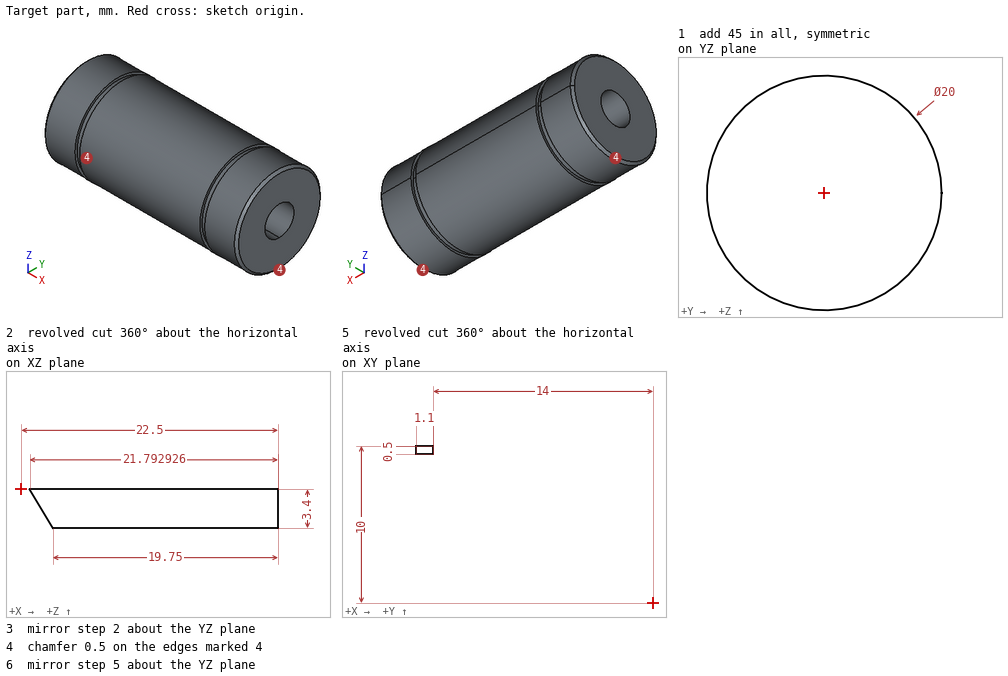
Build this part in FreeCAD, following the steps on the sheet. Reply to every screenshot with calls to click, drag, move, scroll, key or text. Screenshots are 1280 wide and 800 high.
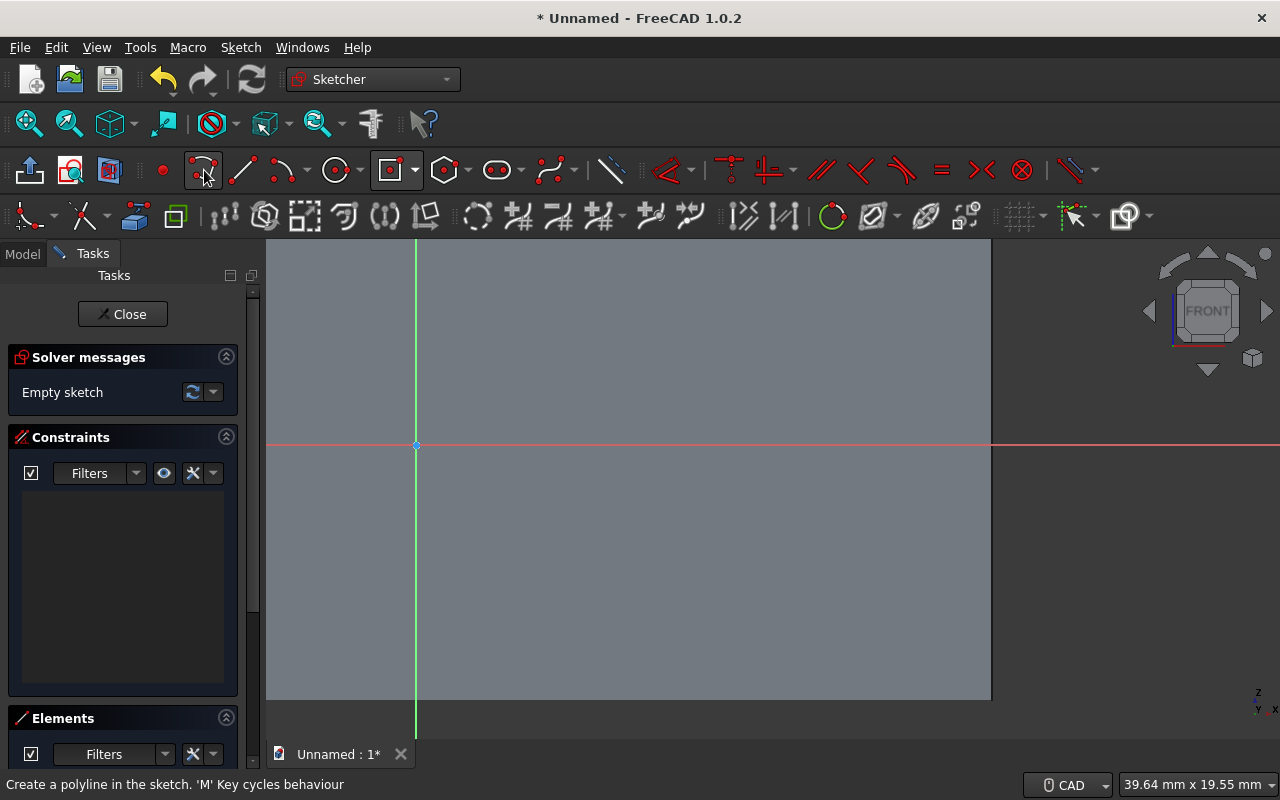
click(434, 445)
click(992, 454)
click(992, 532)
click(486, 532)
click(434, 445)
key(Escape)
key(Escape)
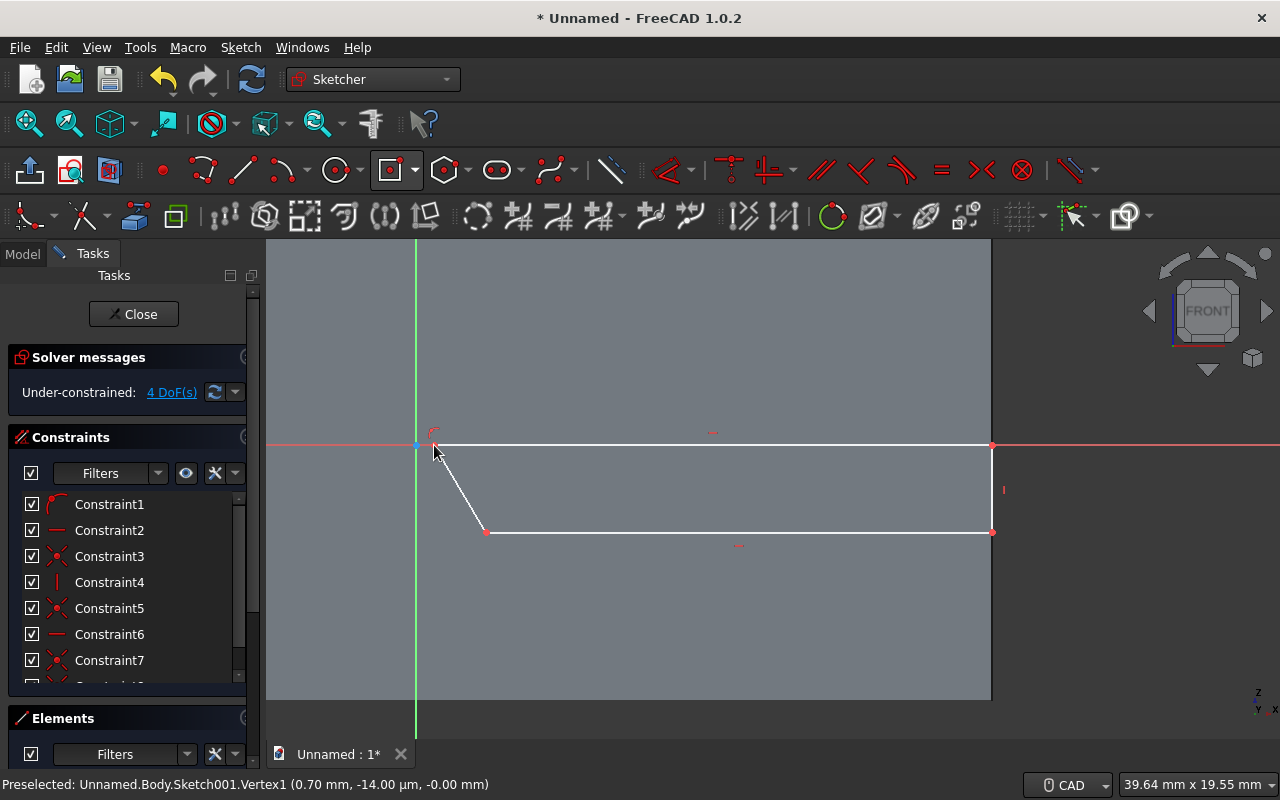
click(992, 471)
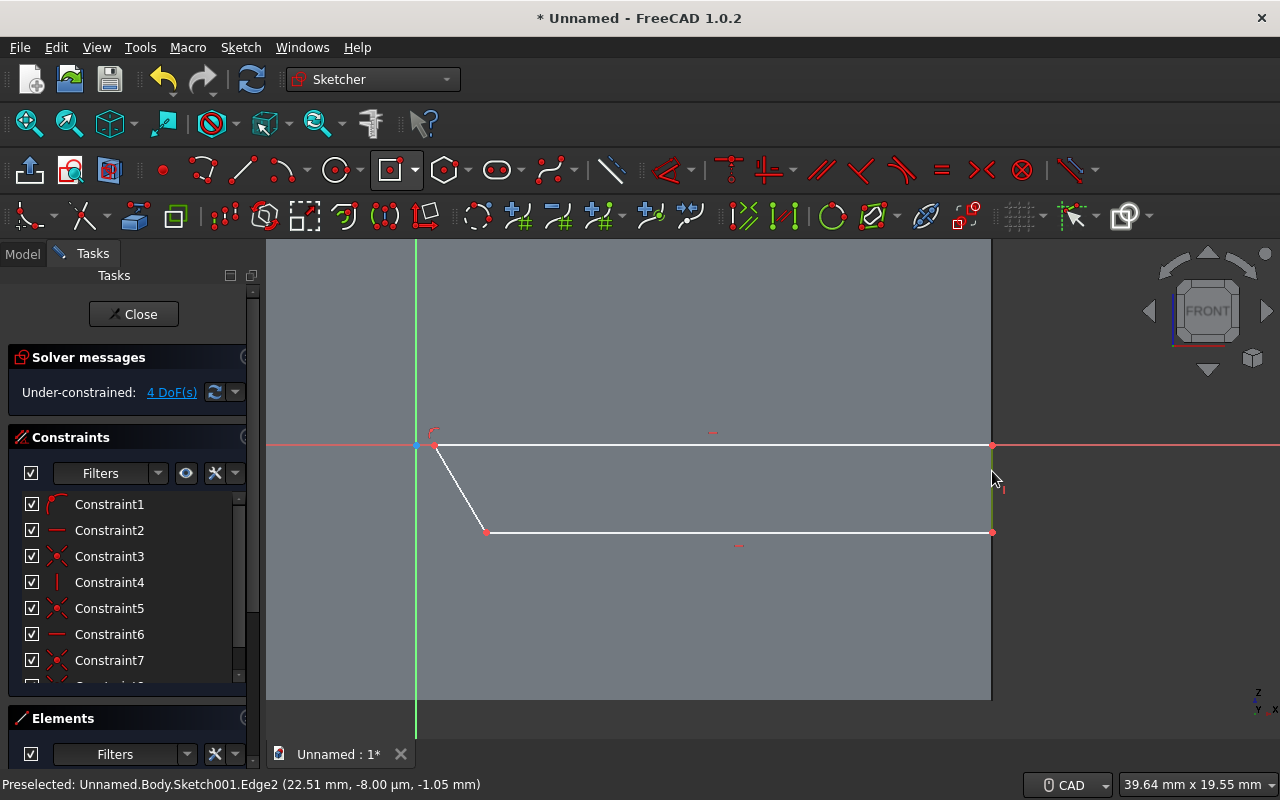
click(694, 170)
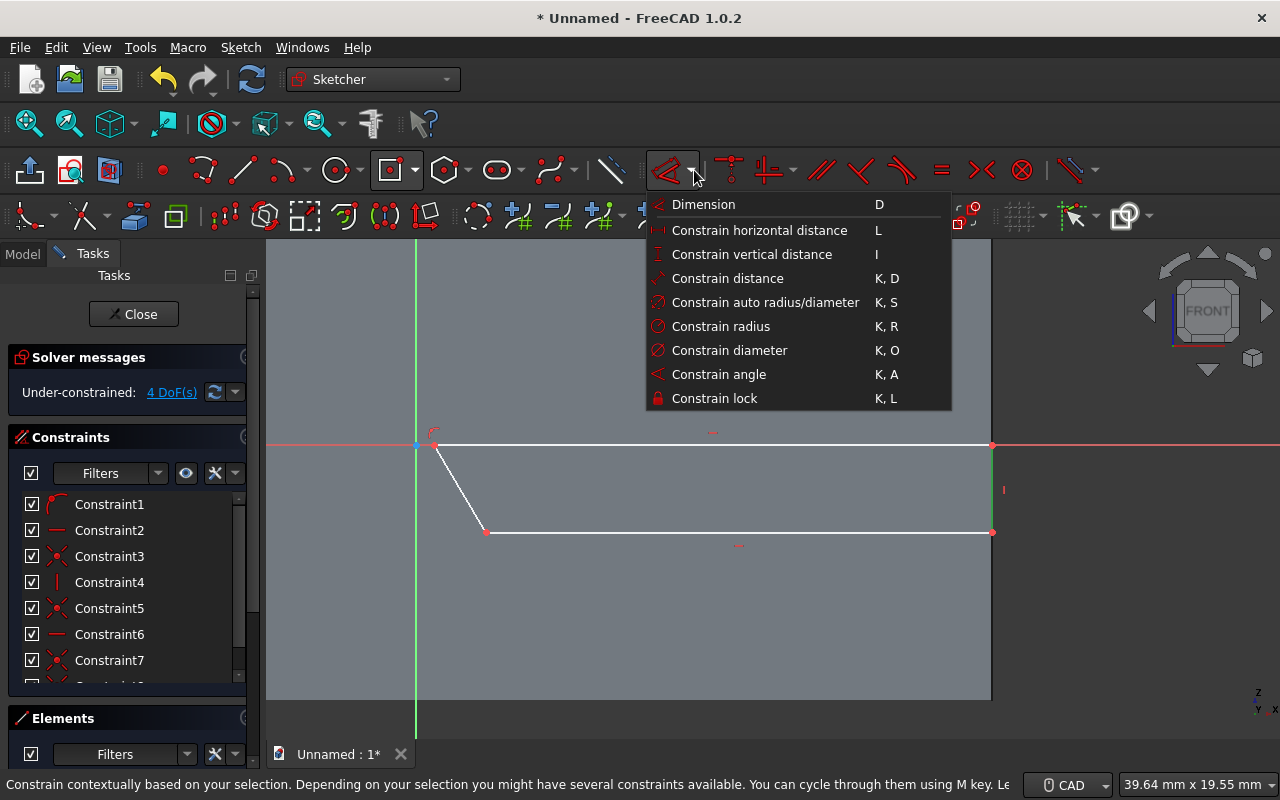
click(799, 254)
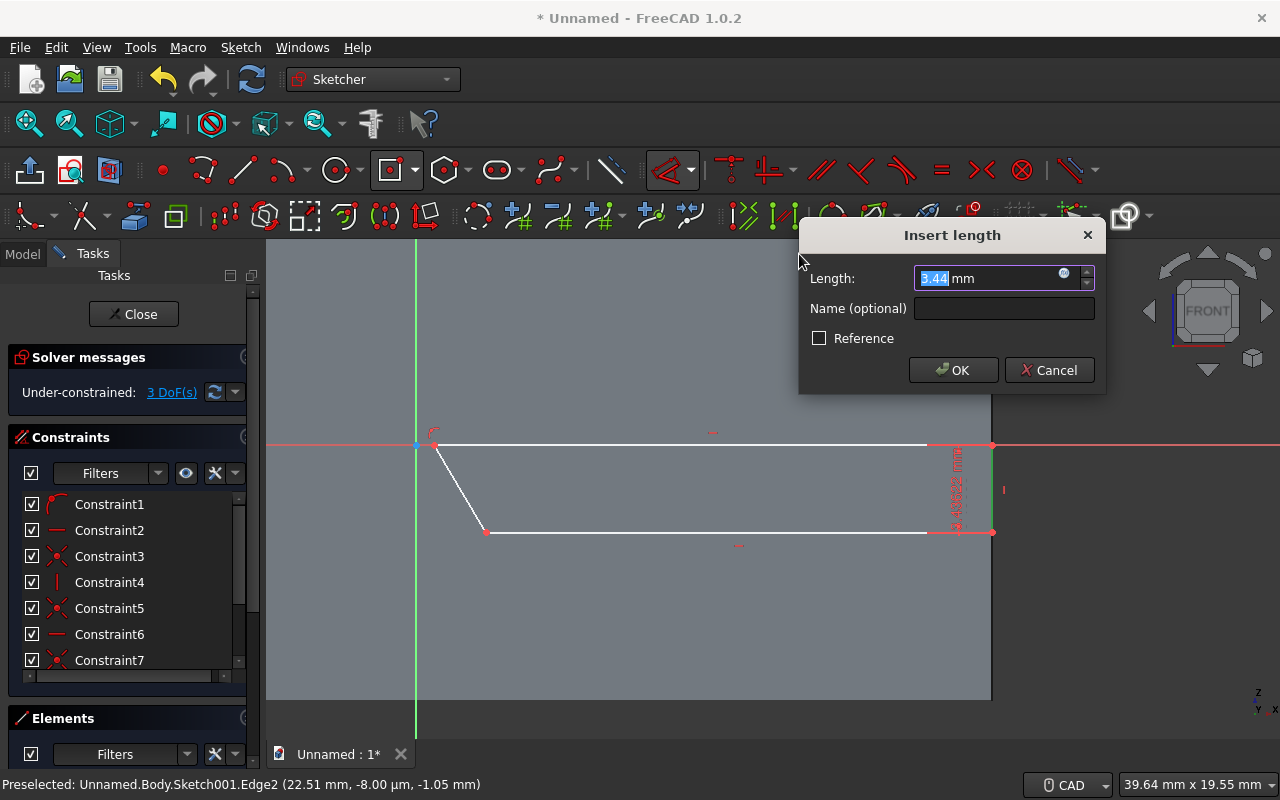
text(3.4)
key(Return)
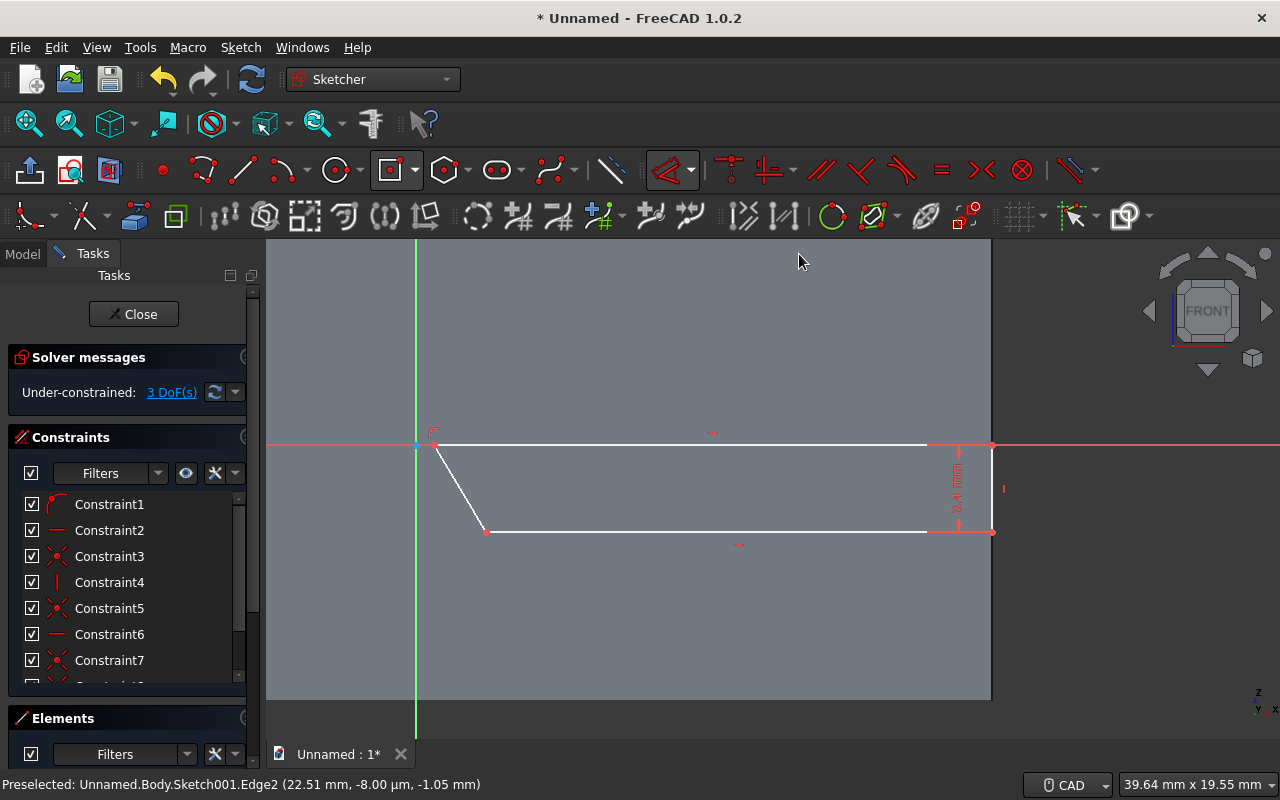
click(840, 532)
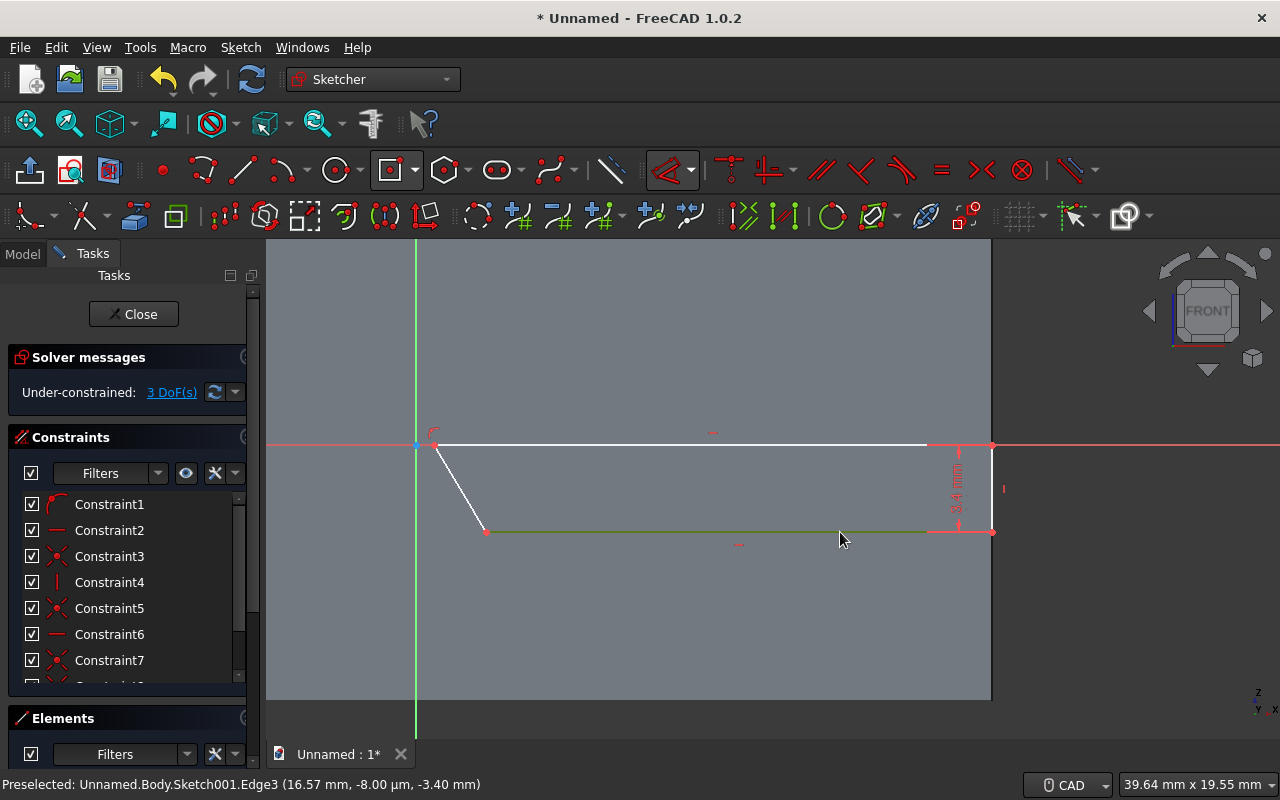
key(l)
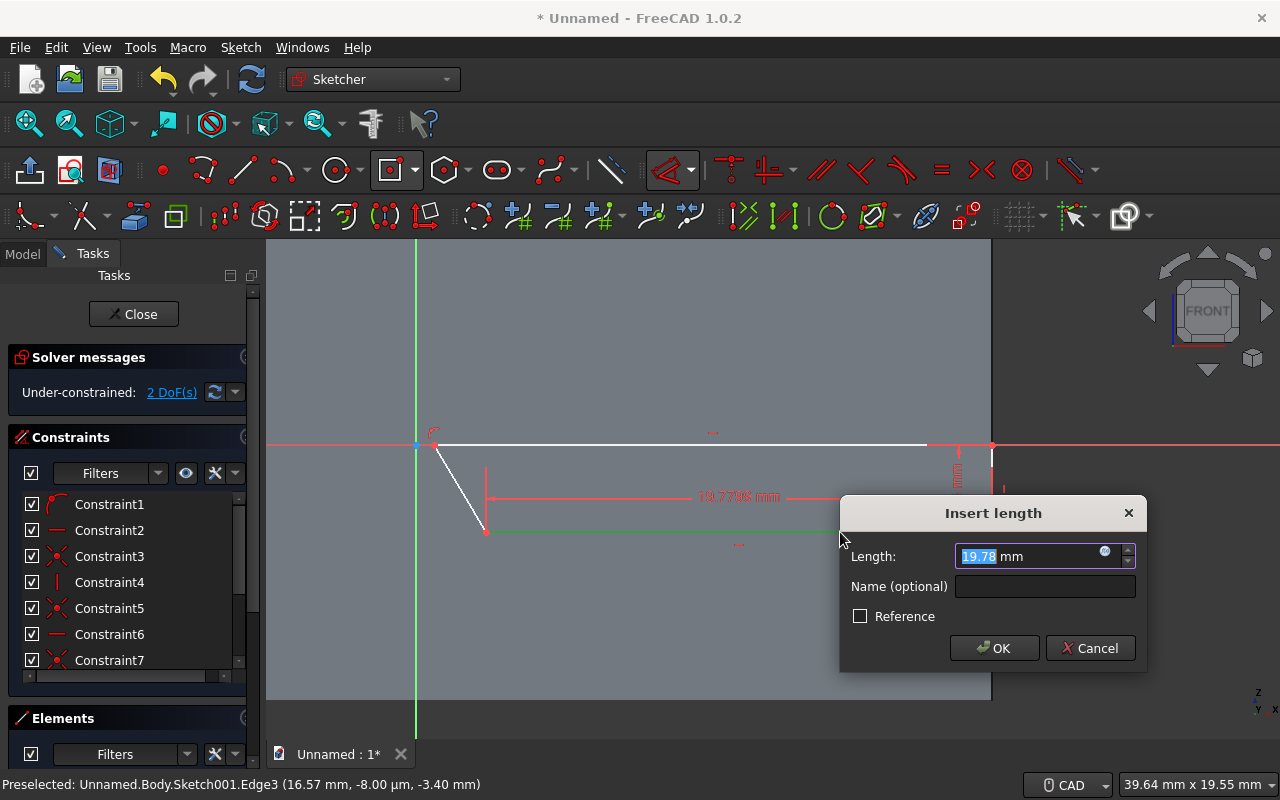
text(19.75)
key(Return)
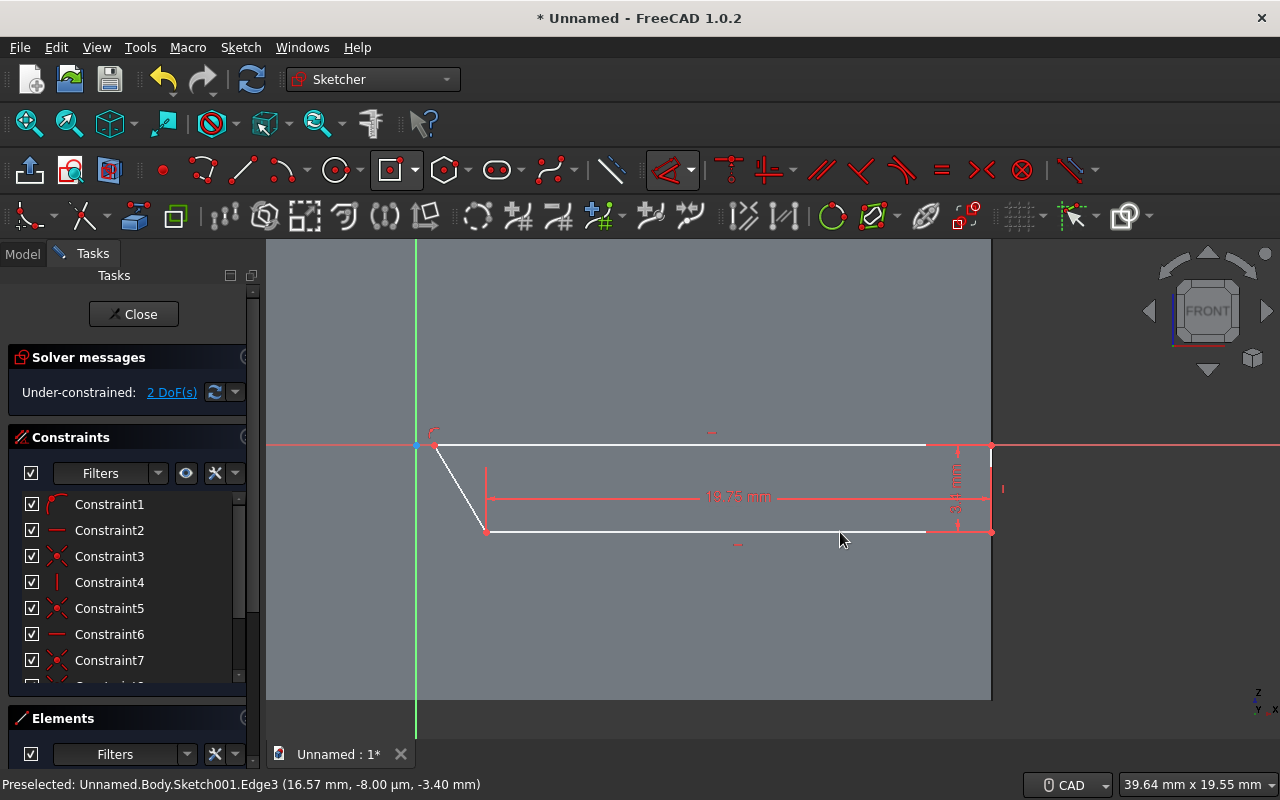
click(991, 445)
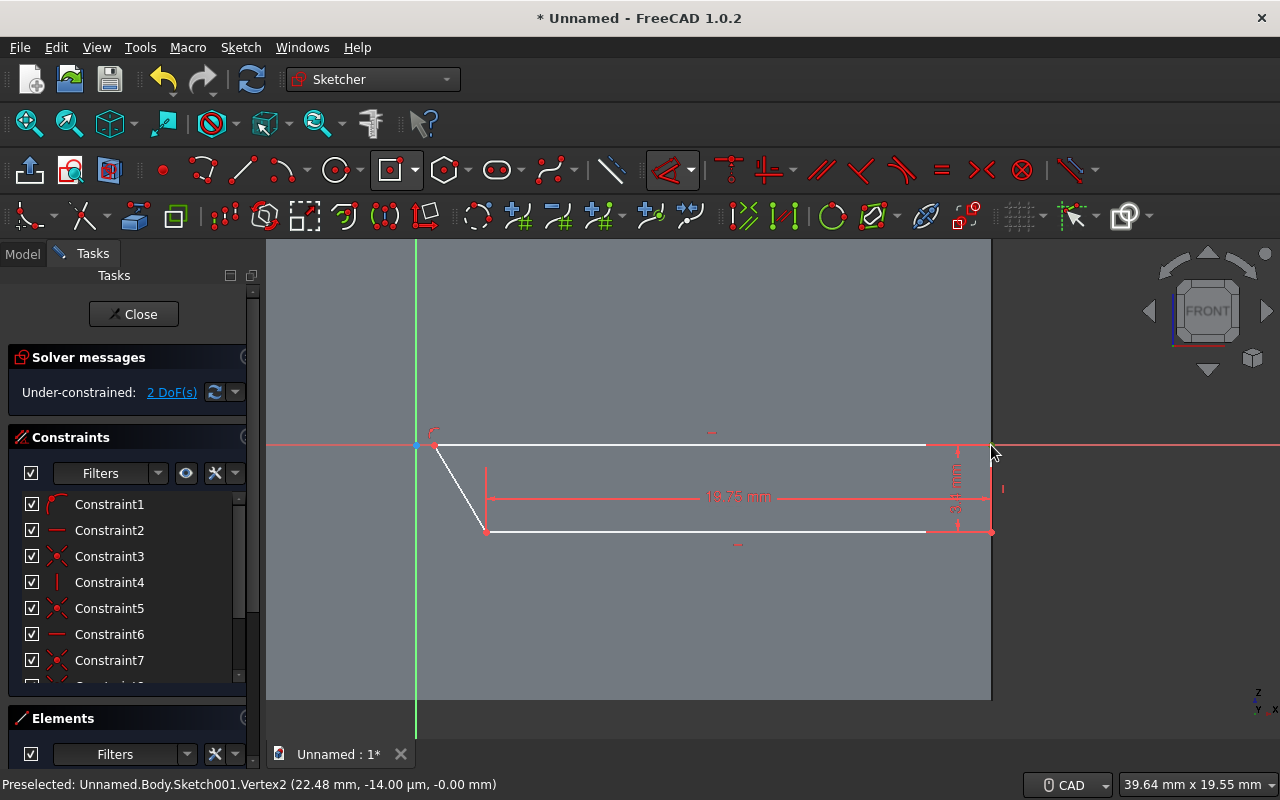
key(l)